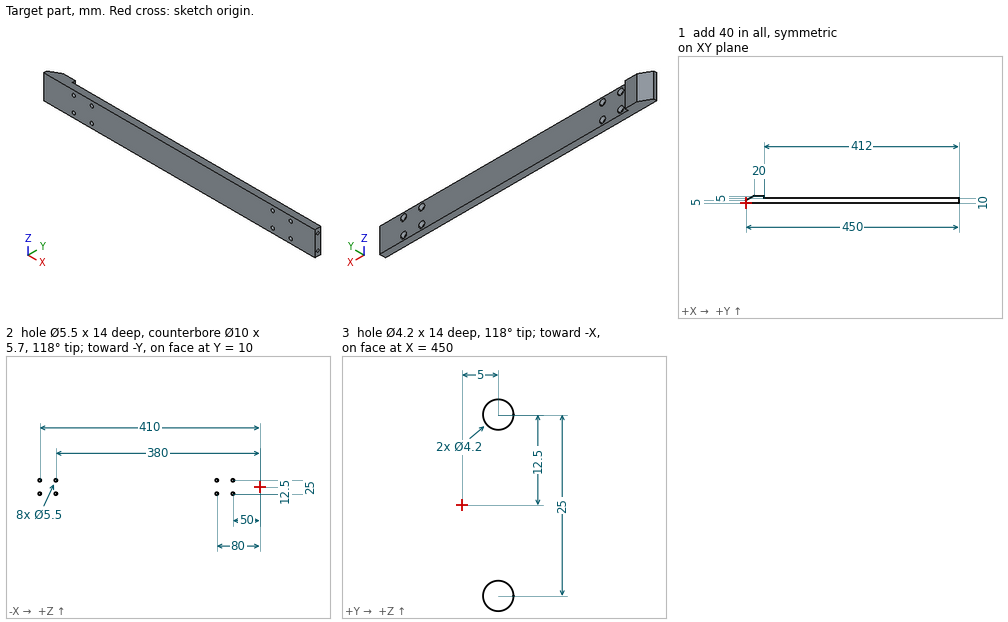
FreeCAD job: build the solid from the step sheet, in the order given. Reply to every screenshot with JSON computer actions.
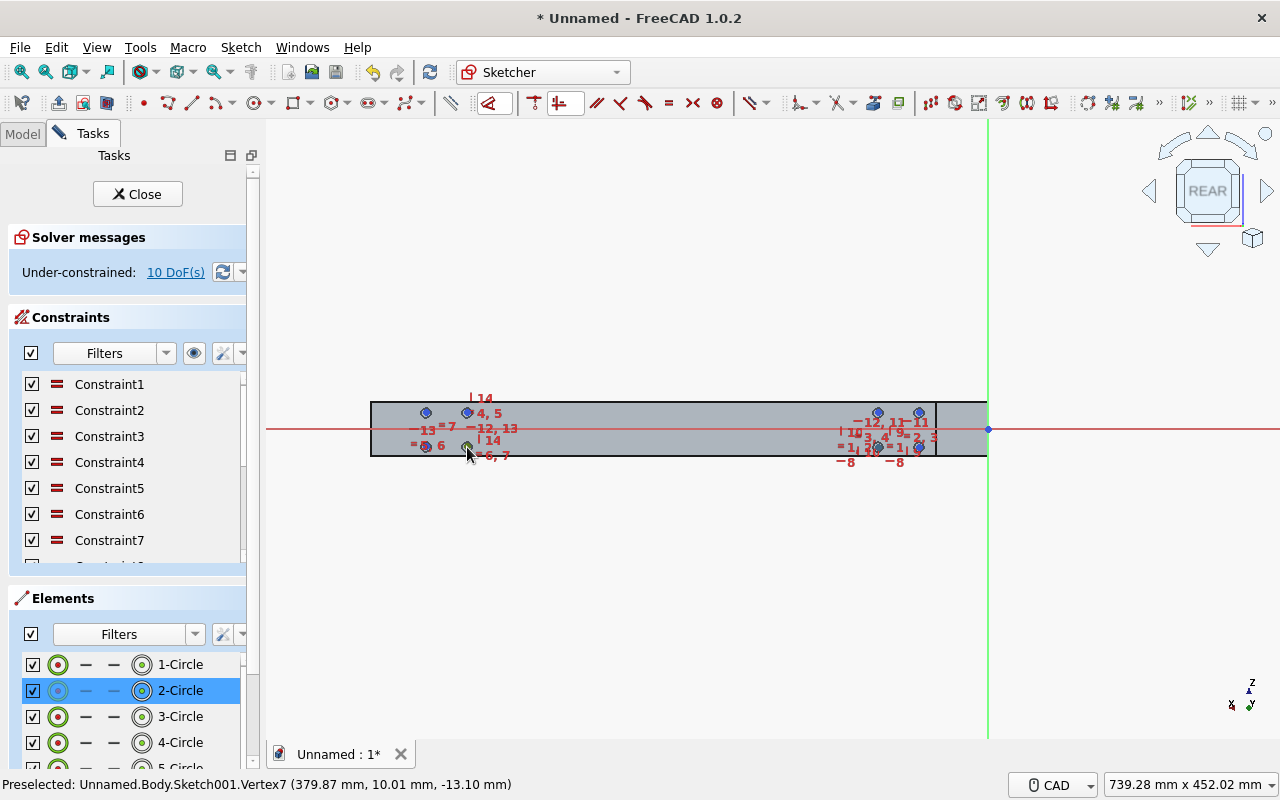
{"action": "key", "text": "h"}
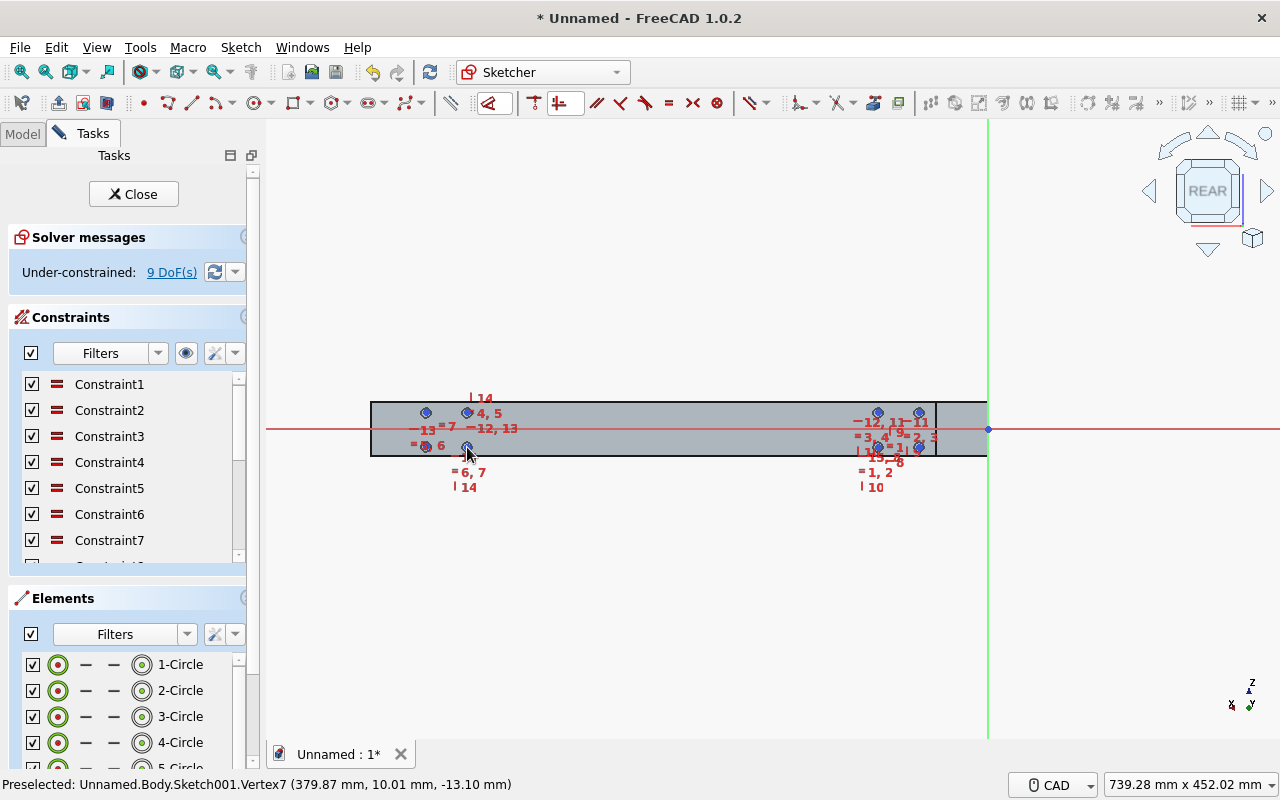
{"action": "left_click", "coordinate": [426, 413]}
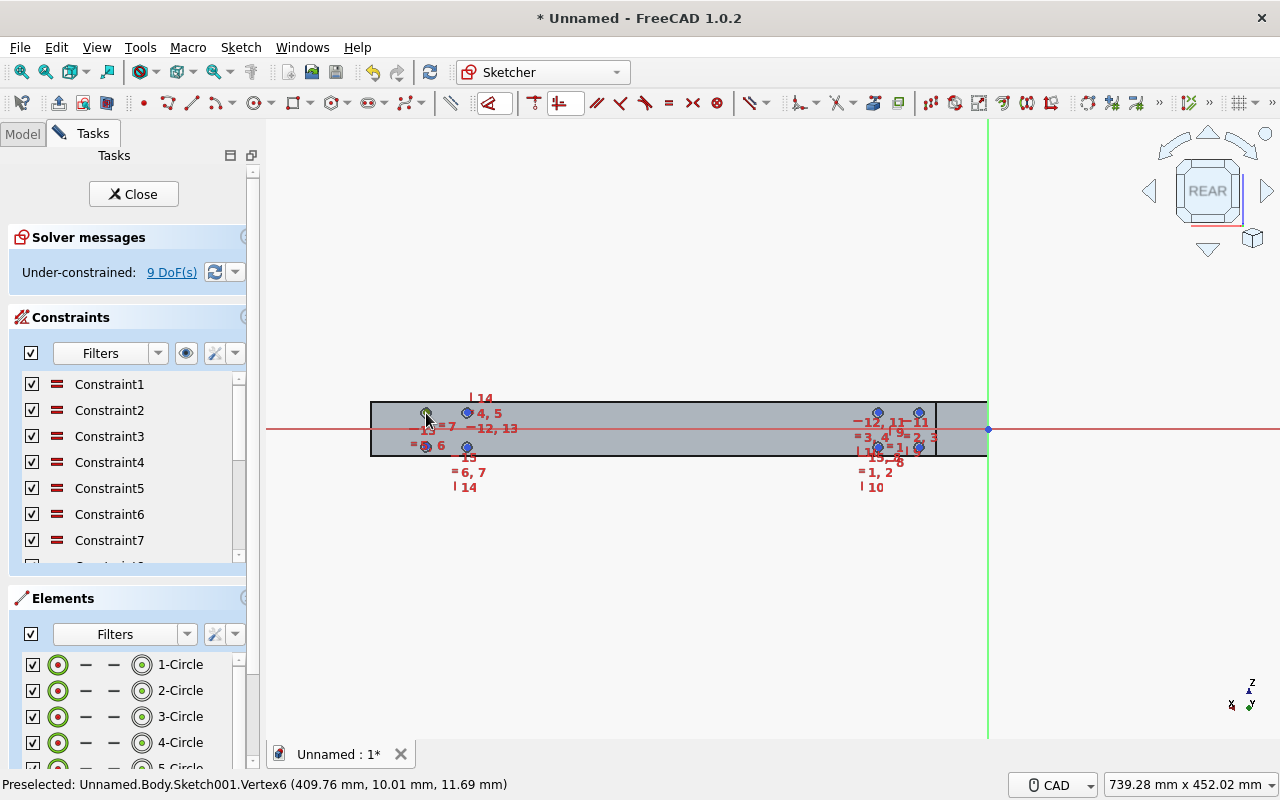
{"action": "scroll", "coordinate": [426, 447], "scroll_direction": "up", "scroll_amount": 4}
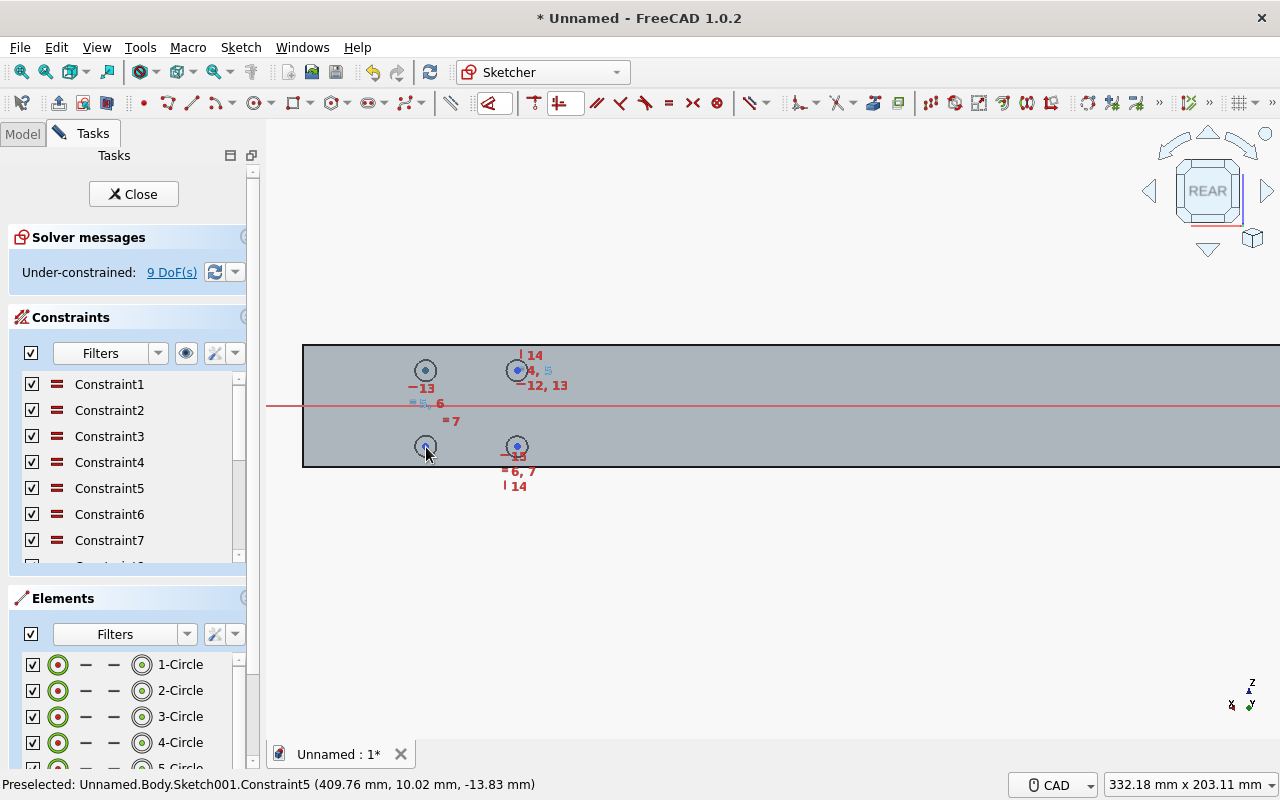
{"action": "left_click", "coordinate": [426, 446]}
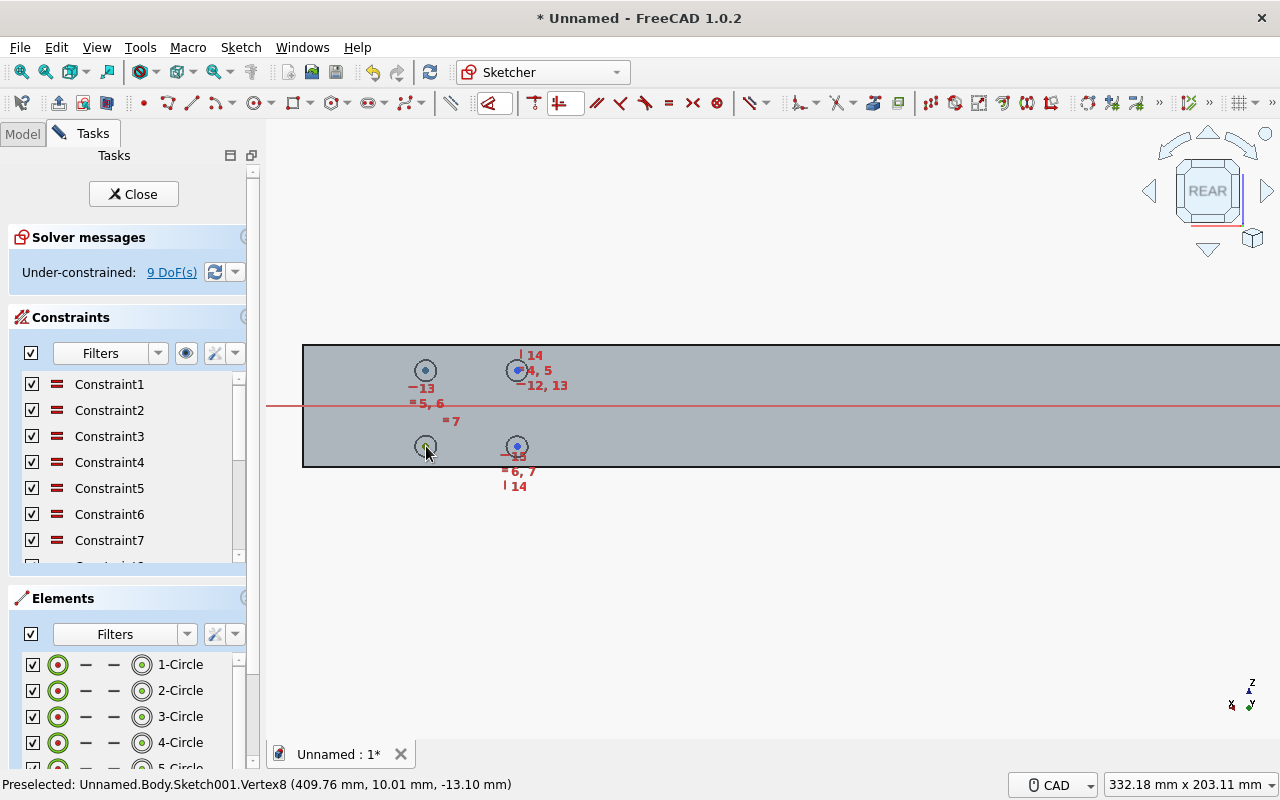
{"action": "key", "text": "v"}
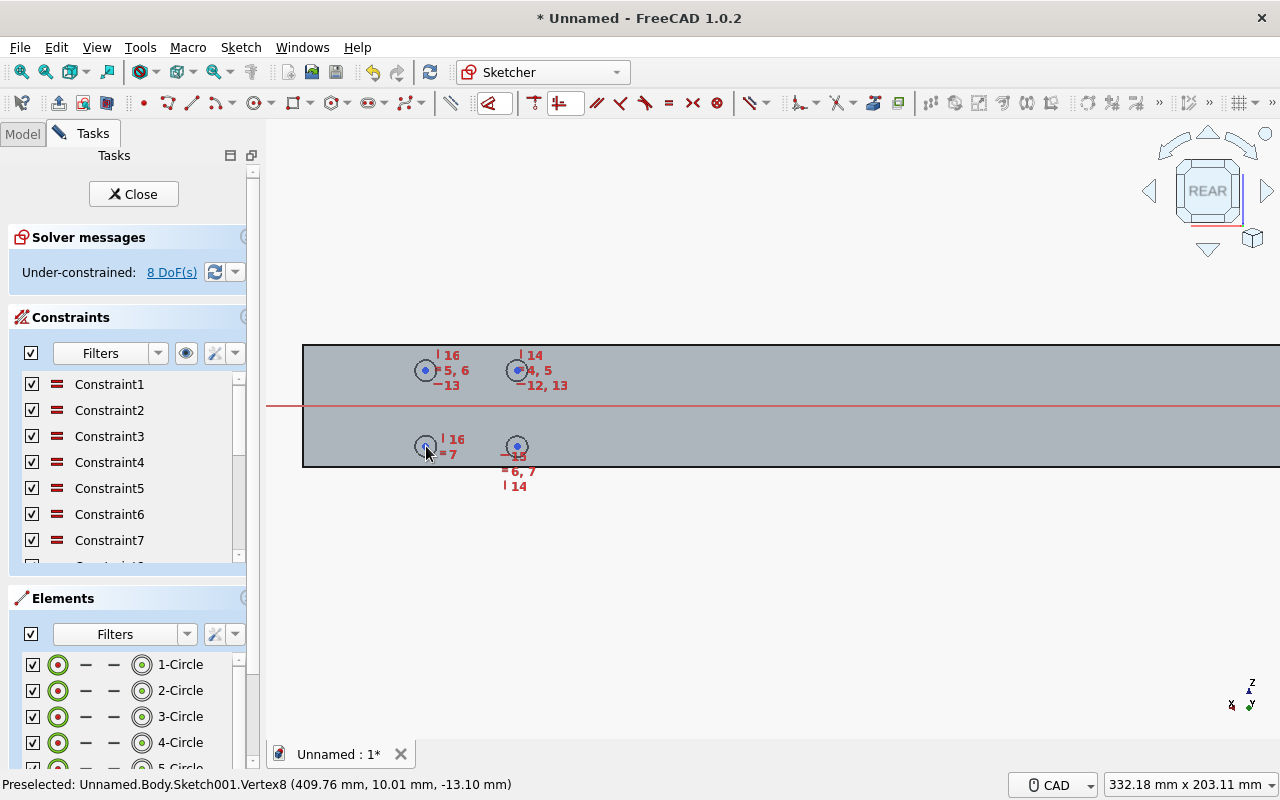
{"action": "left_click", "coordinate": [517, 447]}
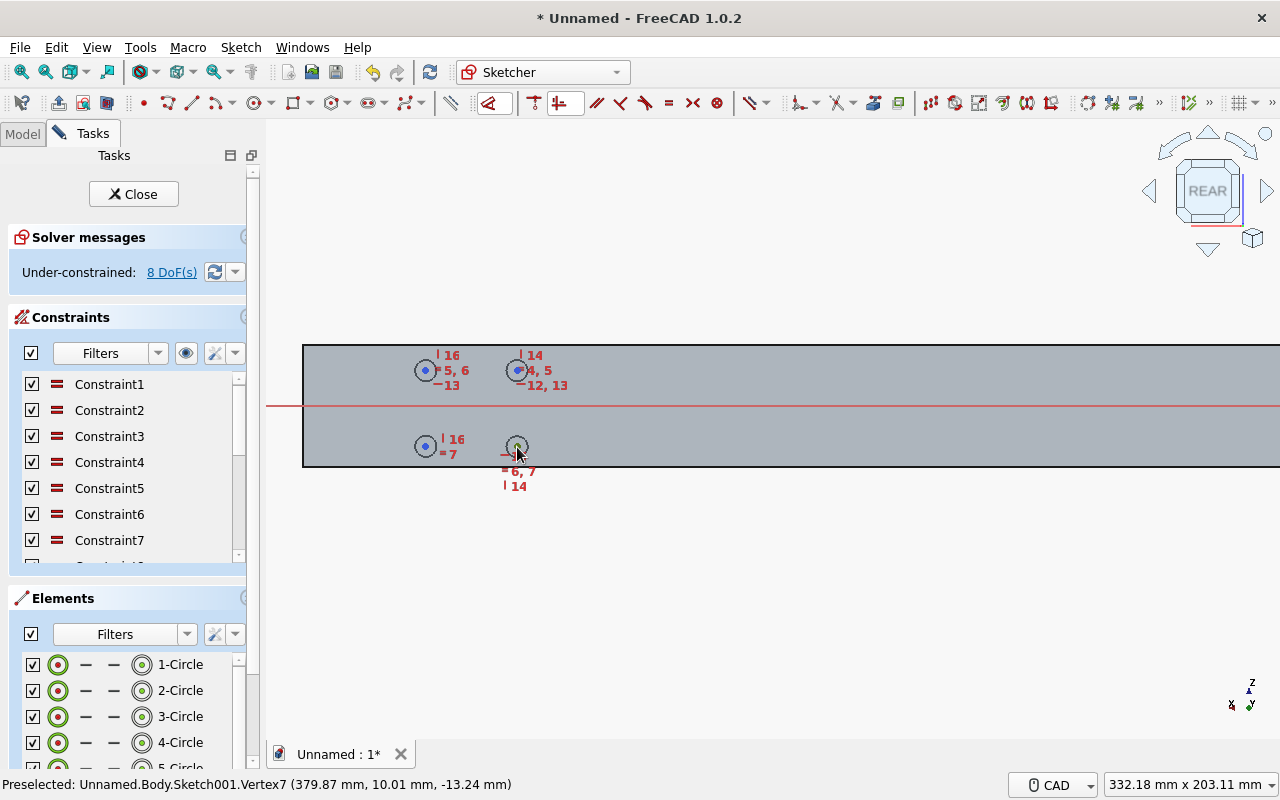
{"action": "left_click", "coordinate": [426, 446]}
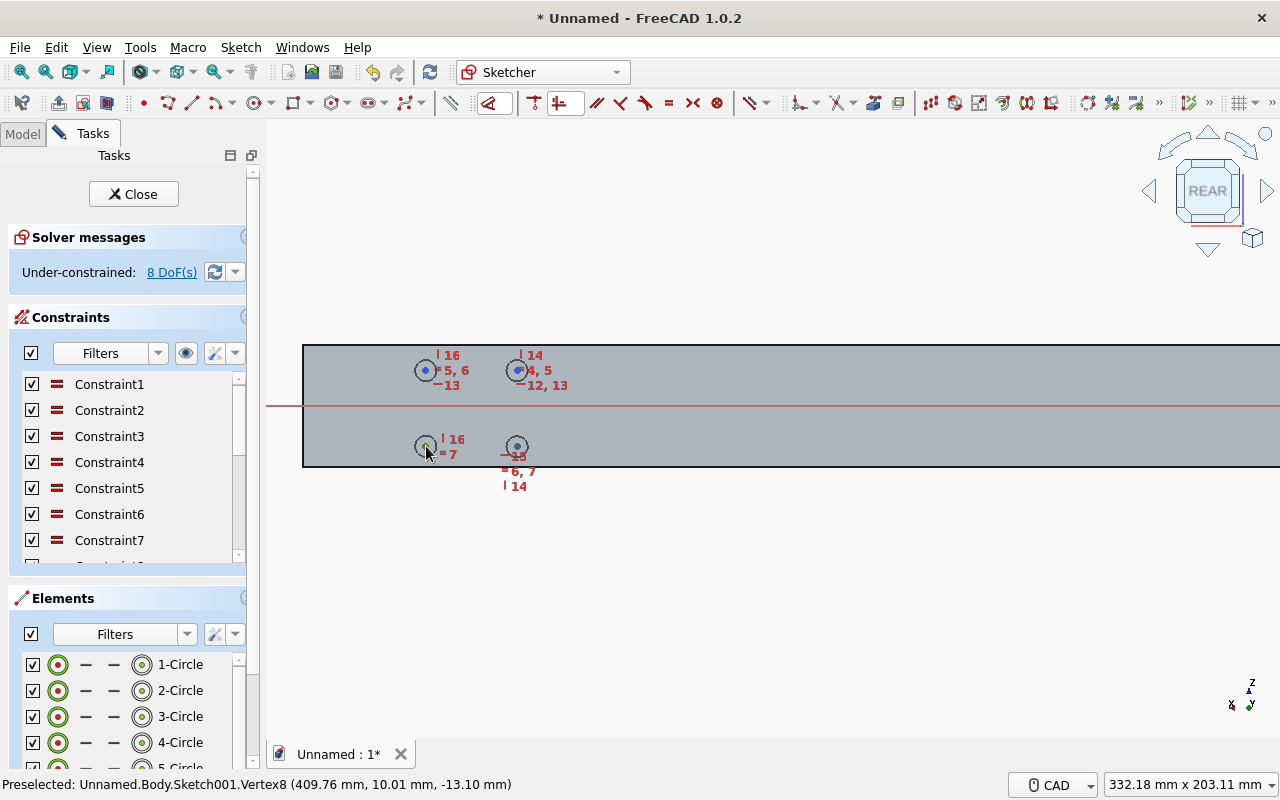
{"action": "left_click", "coordinate": [578, 104]}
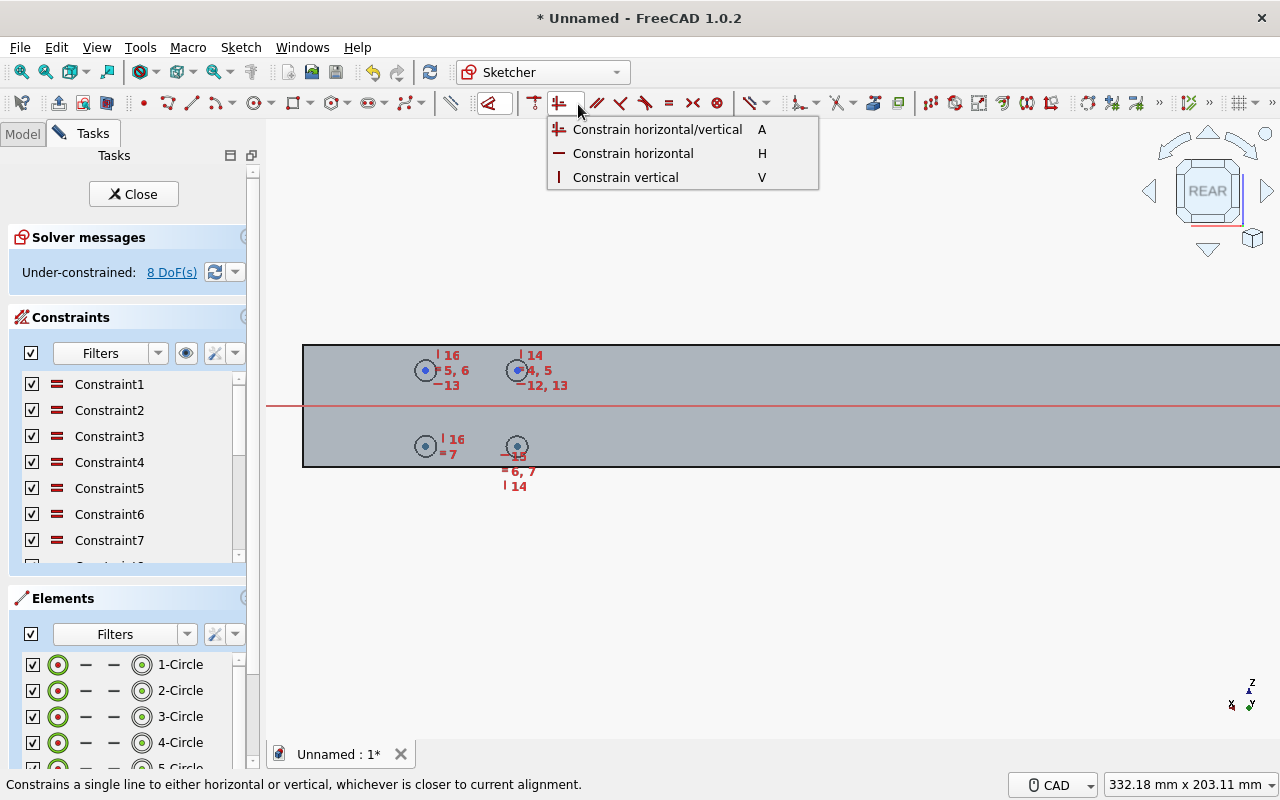
{"action": "left_click", "coordinate": [683, 153]}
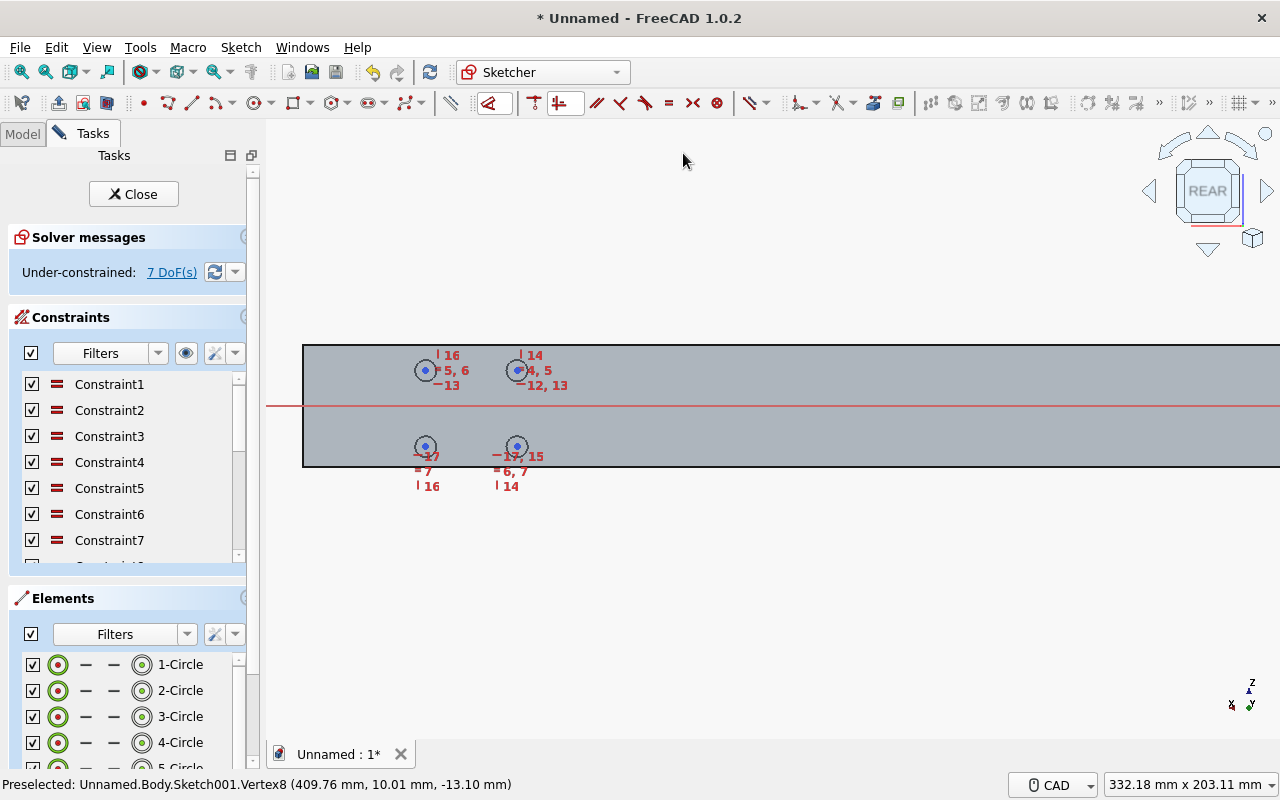
{"action": "scroll", "coordinate": [425, 447], "scroll_direction": "down", "scroll_amount": 4}